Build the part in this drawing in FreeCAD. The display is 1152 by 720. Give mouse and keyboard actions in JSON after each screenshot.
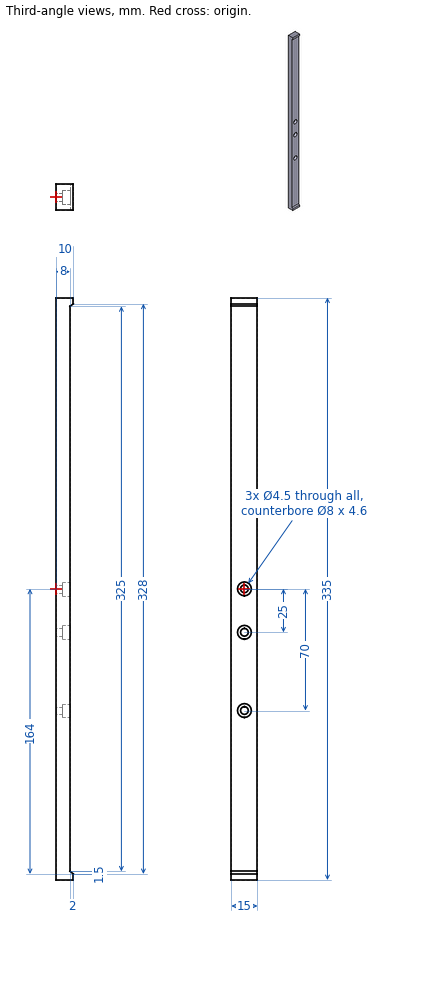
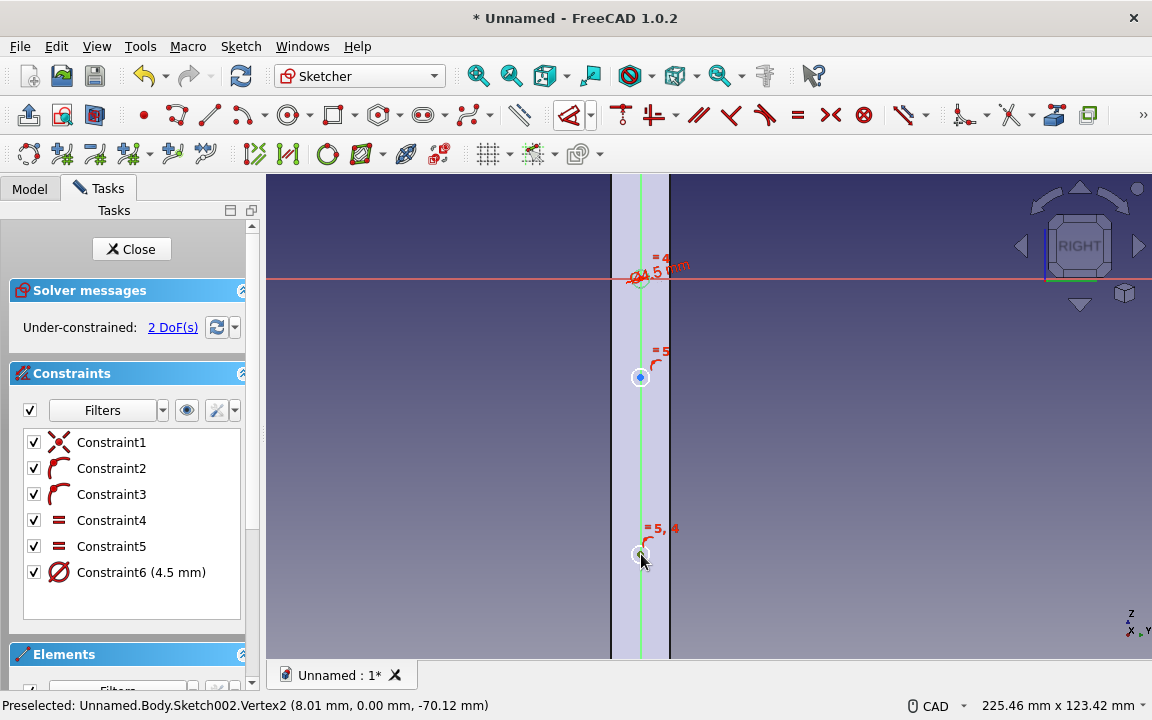
{"action": "key", "text": "i"}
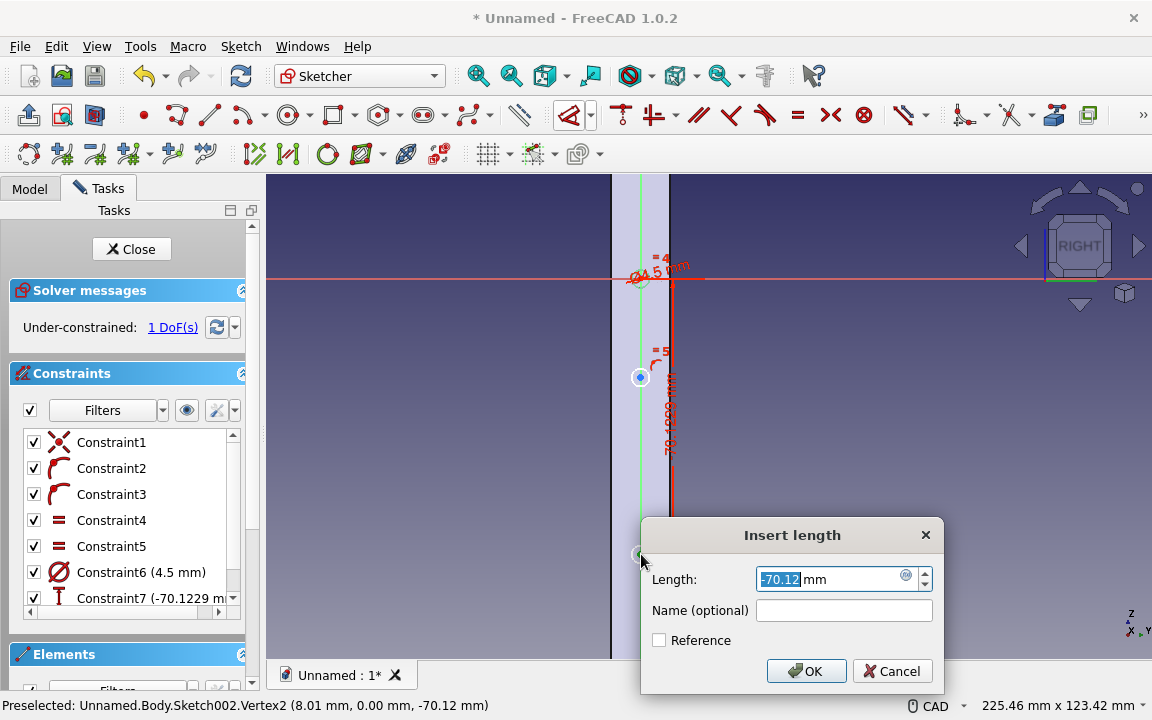
{"action": "type", "text": "-70"}
{"action": "key", "text": "Return"}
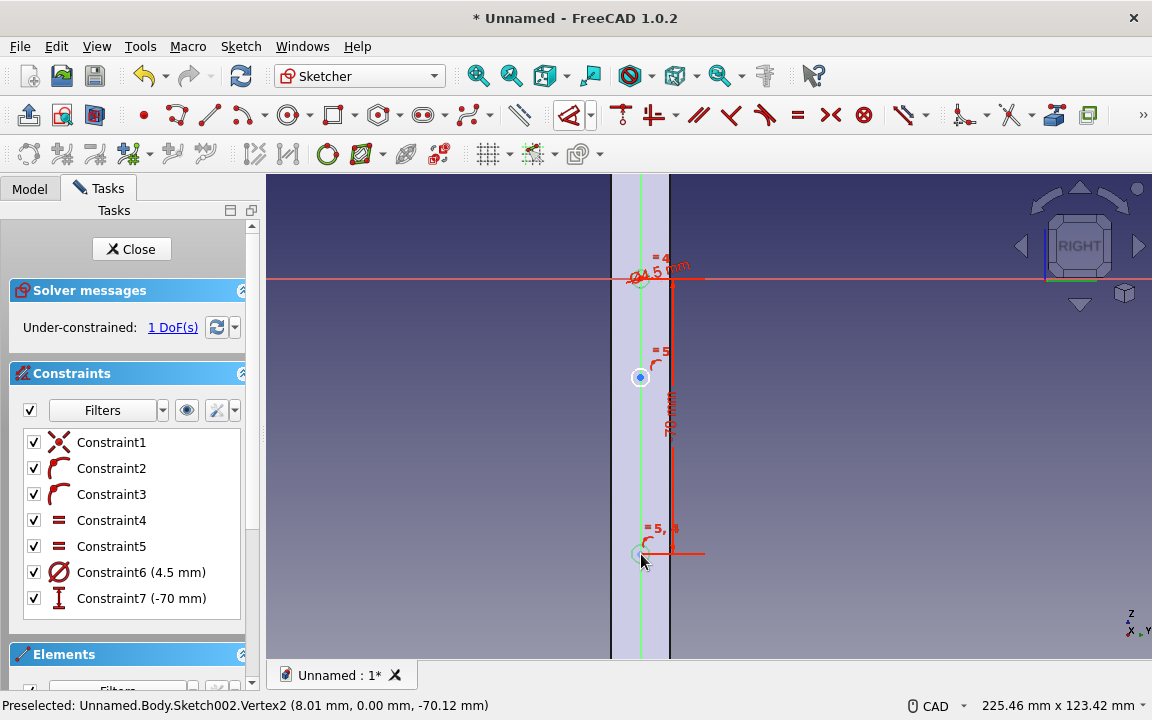
{"action": "left_click", "coordinate": [641, 378]}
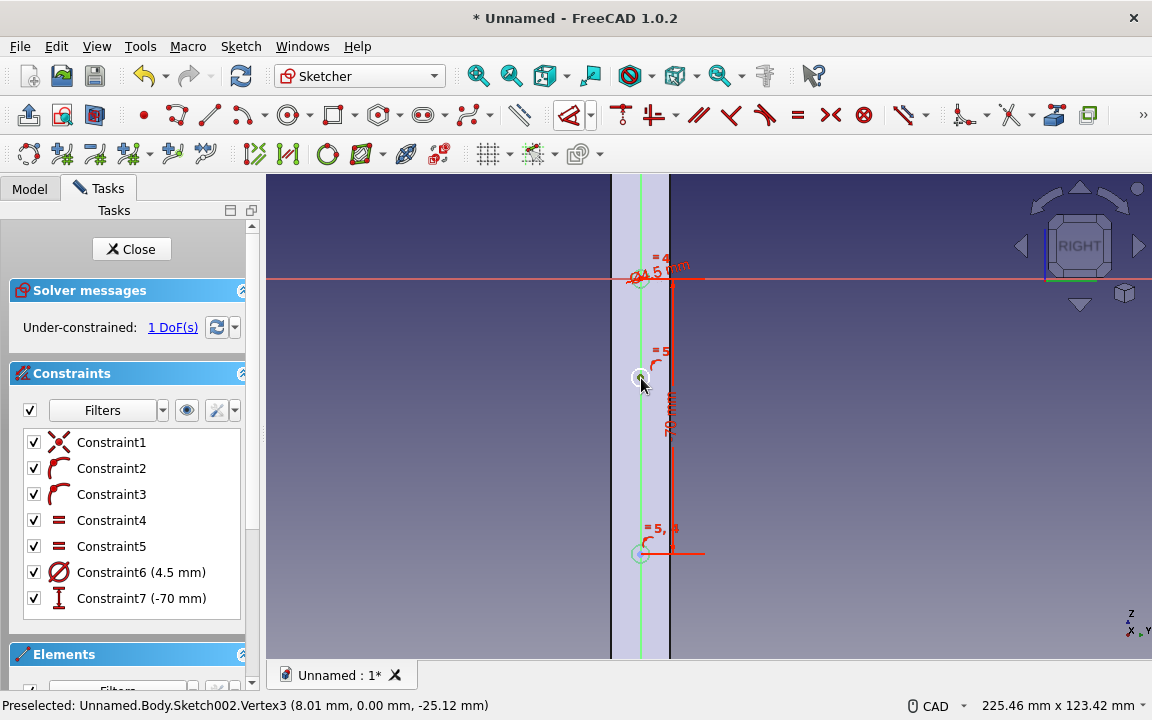
{"action": "left_click", "coordinate": [590, 116]}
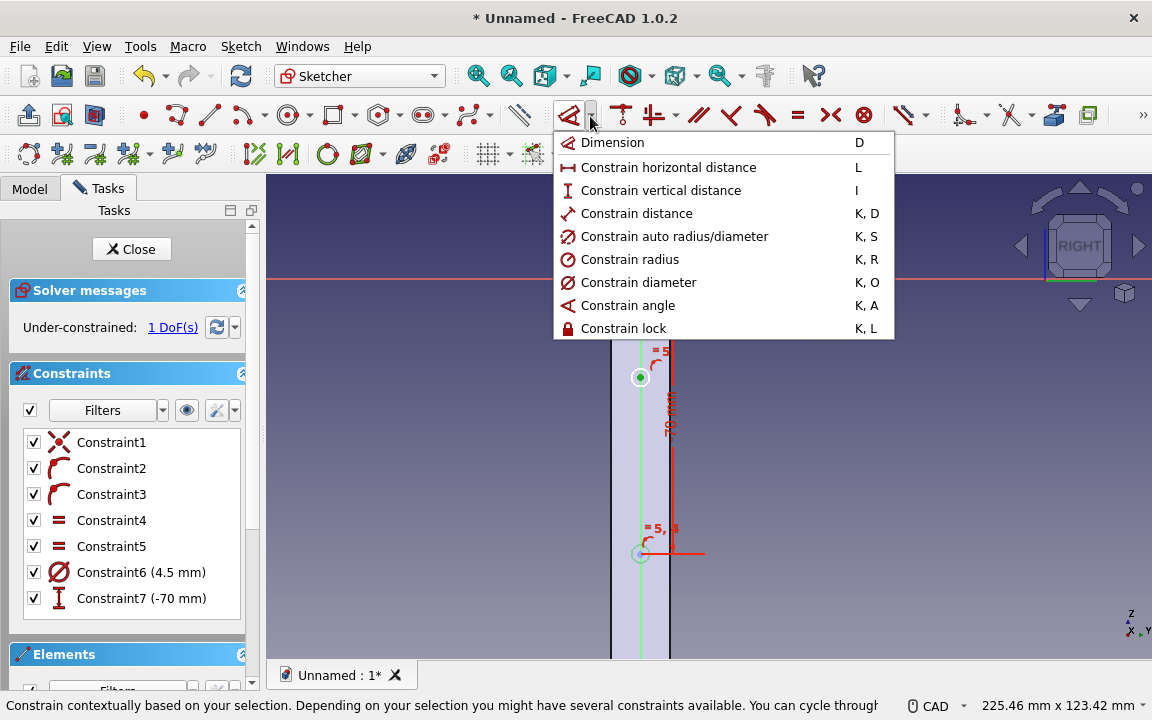
{"action": "left_click", "coordinate": [724, 190]}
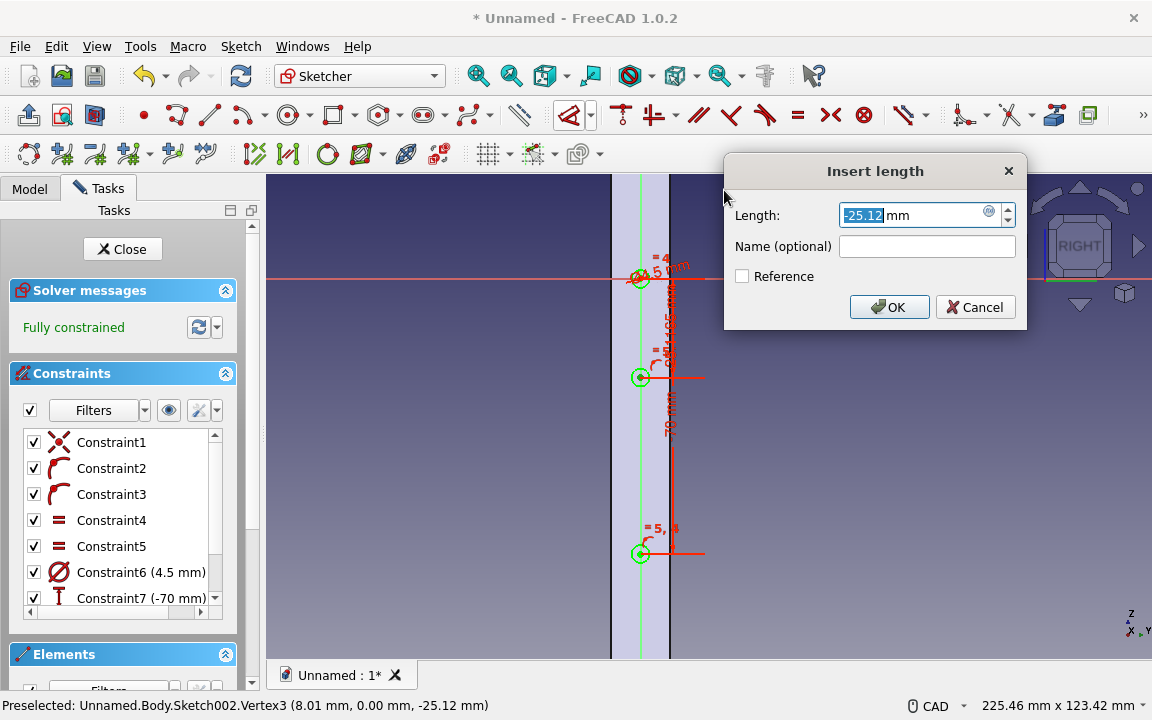
{"action": "type", "text": "-25"}
{"action": "key", "text": "Return"}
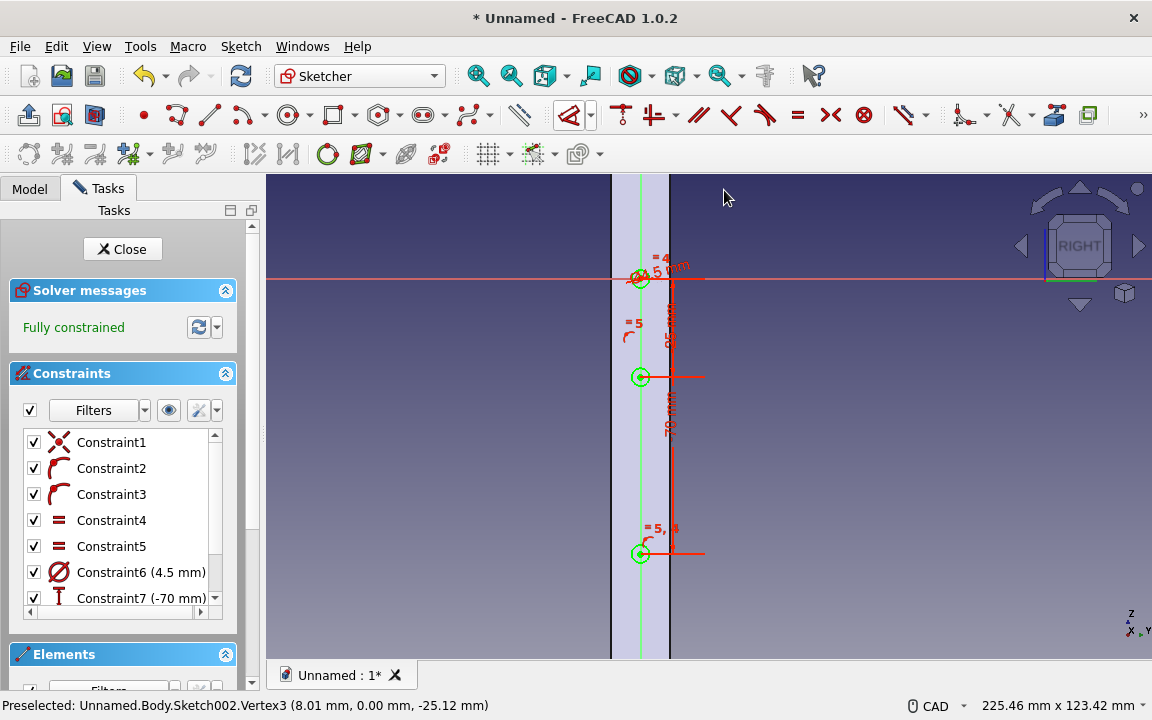
{"action": "left_click", "coordinate": [123, 249]}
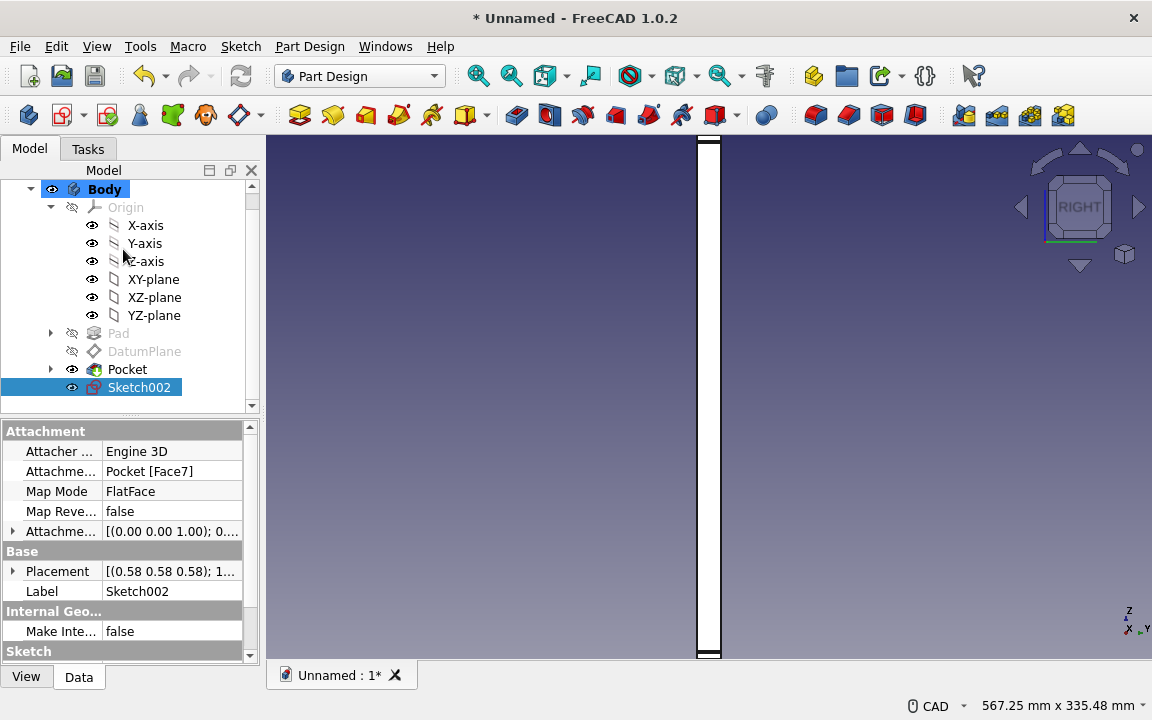
{"action": "left_click", "coordinate": [550, 116]}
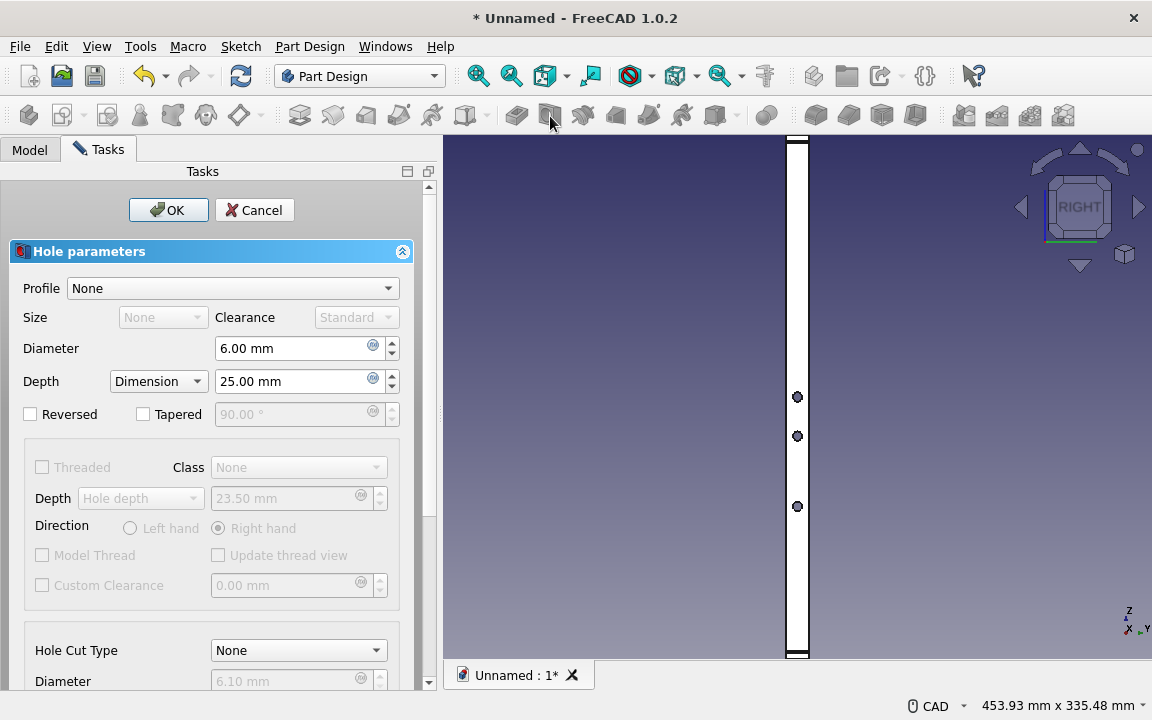
{"action": "triple_click", "coordinate": [300, 348]}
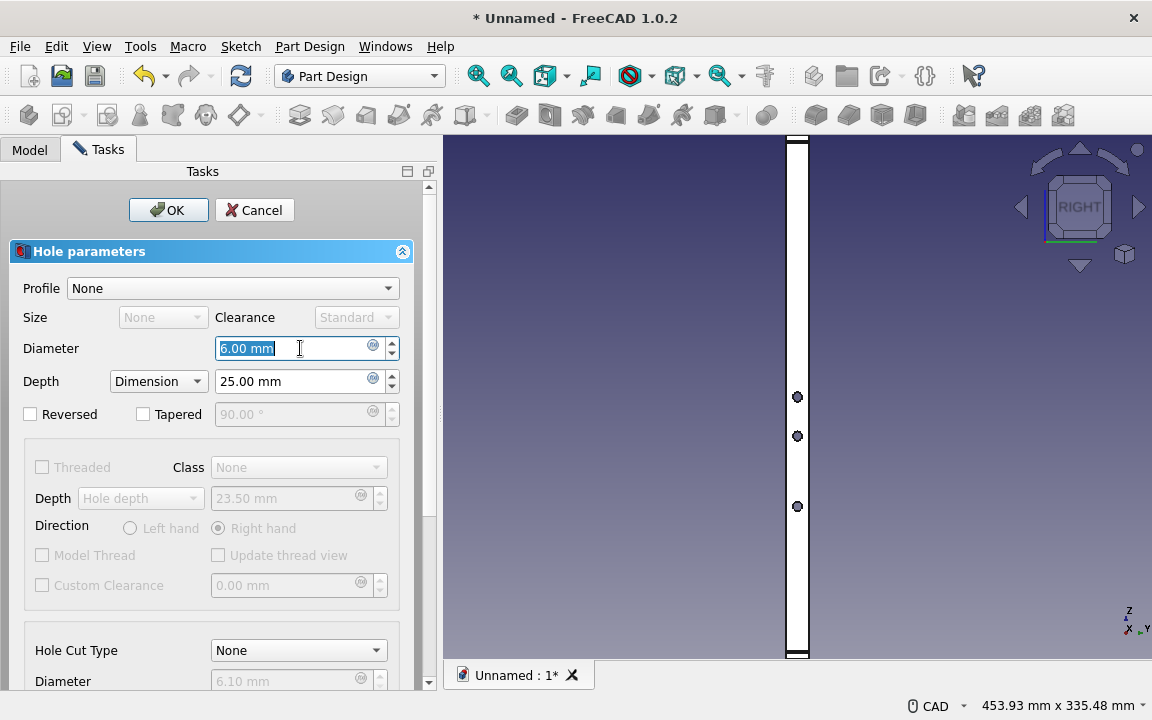
{"action": "type", "text": "4.5"}
{"action": "key", "text": "Tab"}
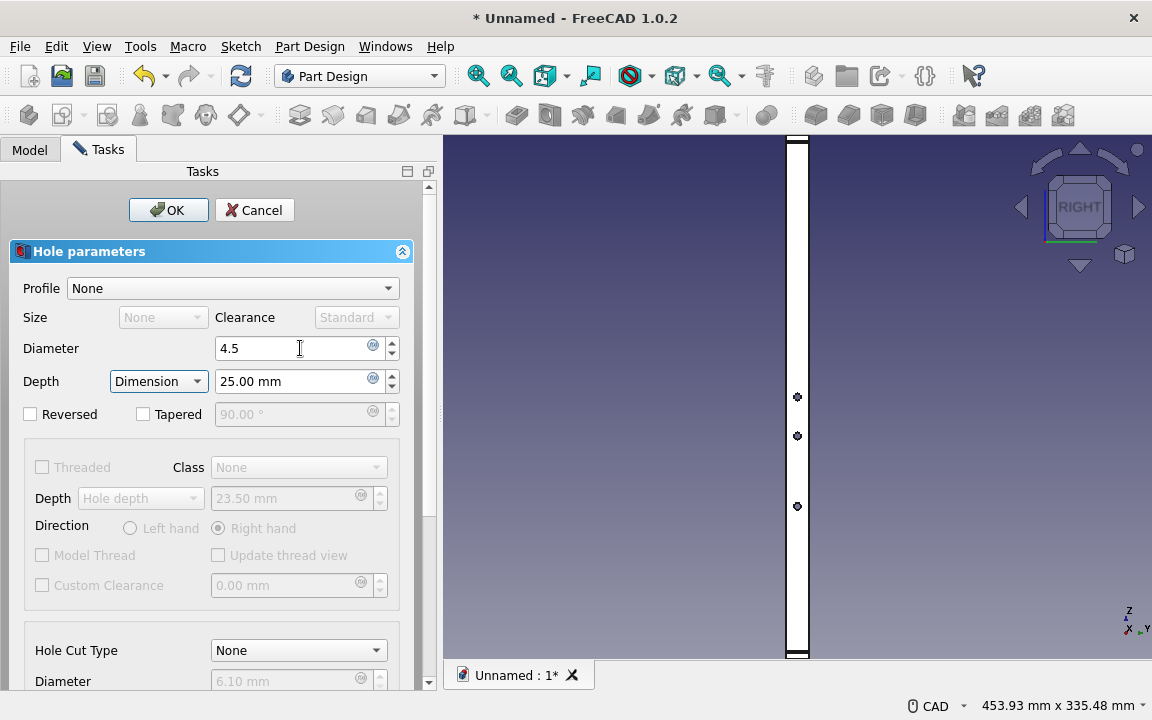
{"action": "left_click", "coordinate": [160, 382]}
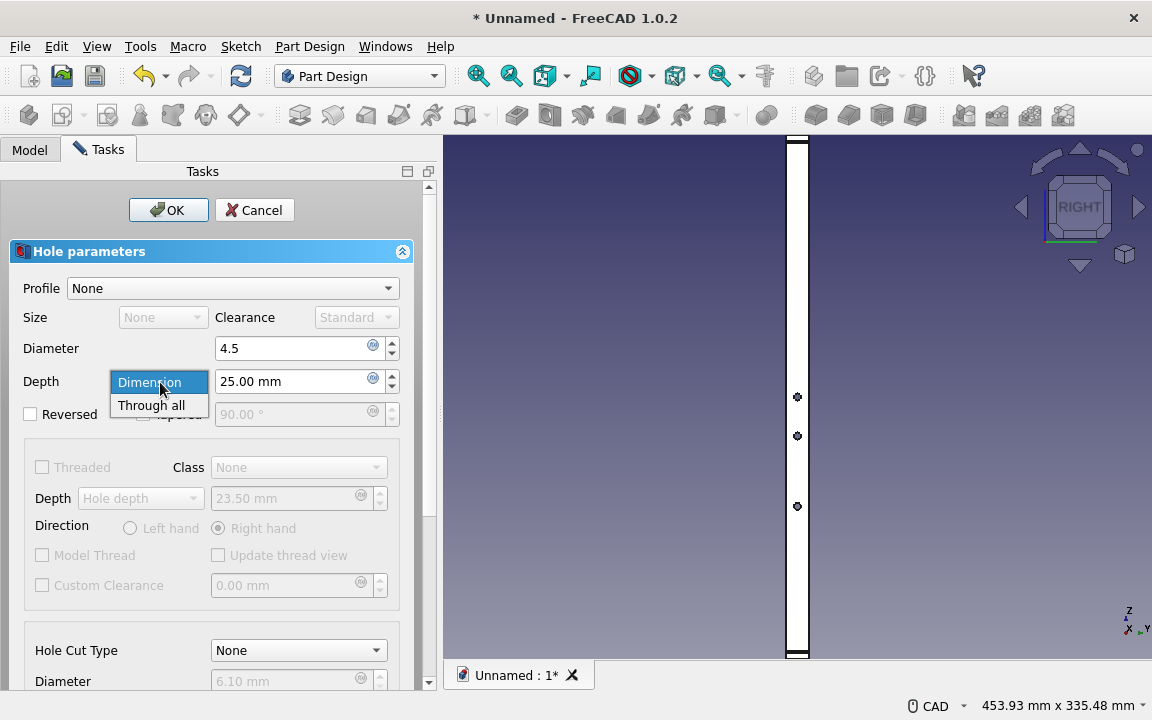
{"action": "left_click", "coordinate": [158, 406]}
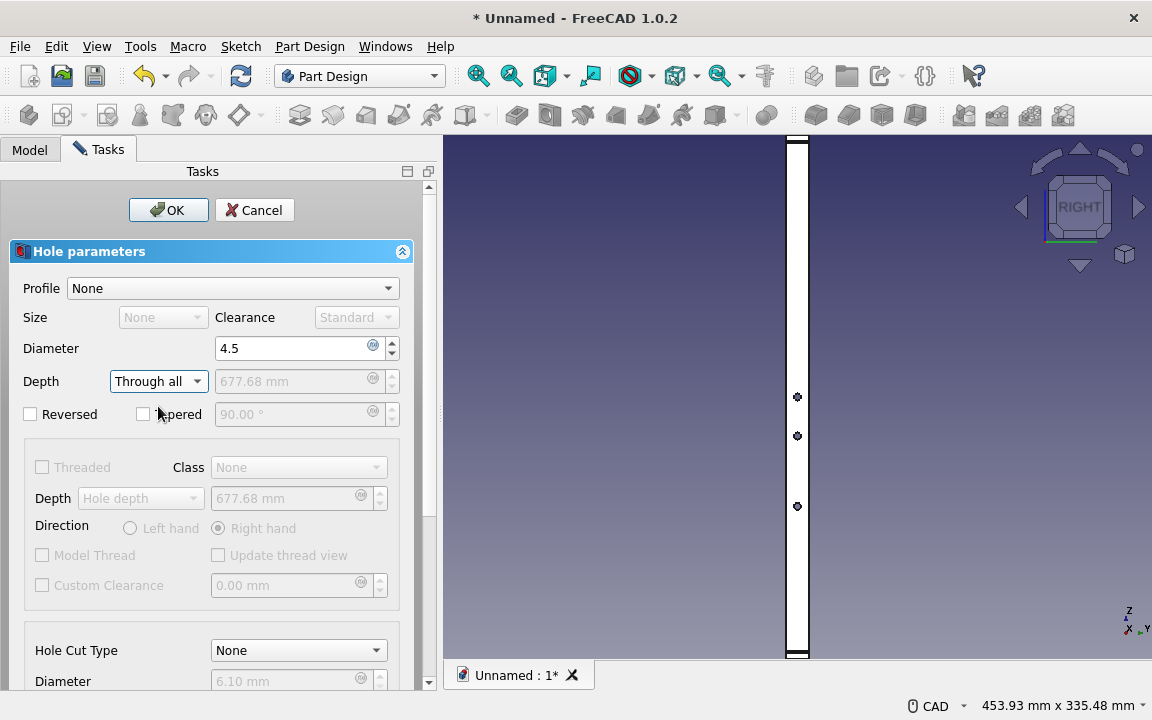
{"action": "left_click", "coordinate": [300, 650]}